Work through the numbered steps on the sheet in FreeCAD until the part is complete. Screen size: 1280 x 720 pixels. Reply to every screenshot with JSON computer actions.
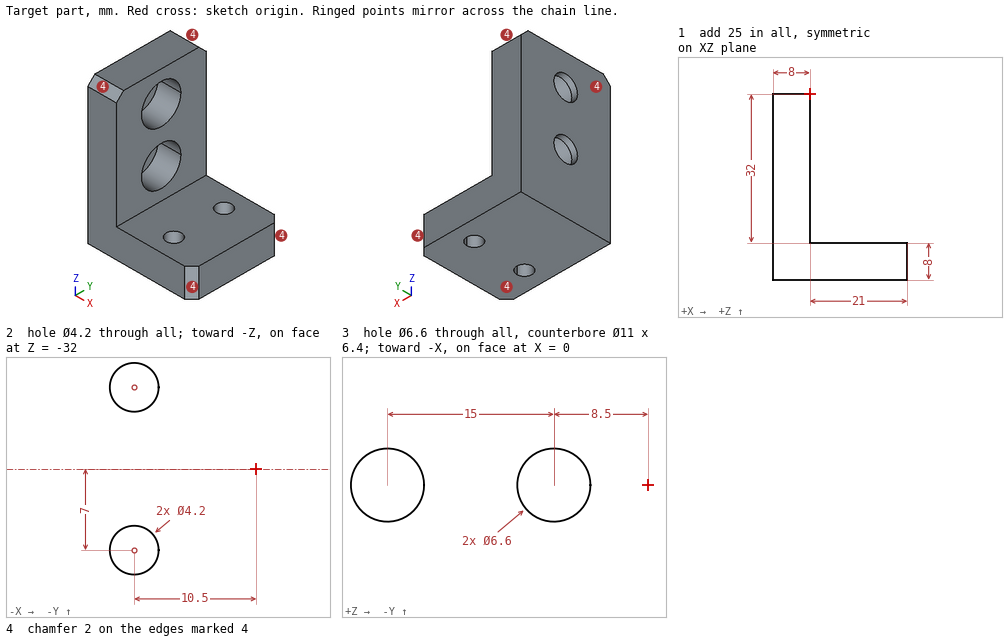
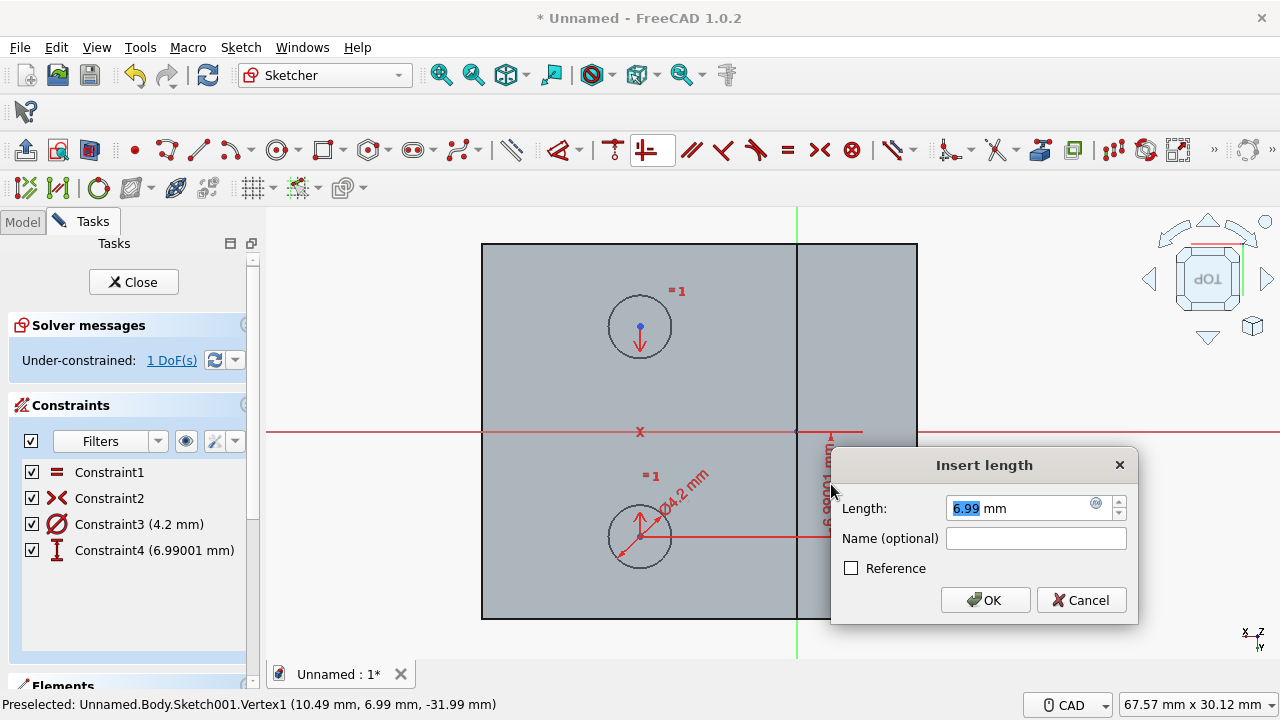
{"action": "type", "text": "7"}
{"action": "key", "text": "Return"}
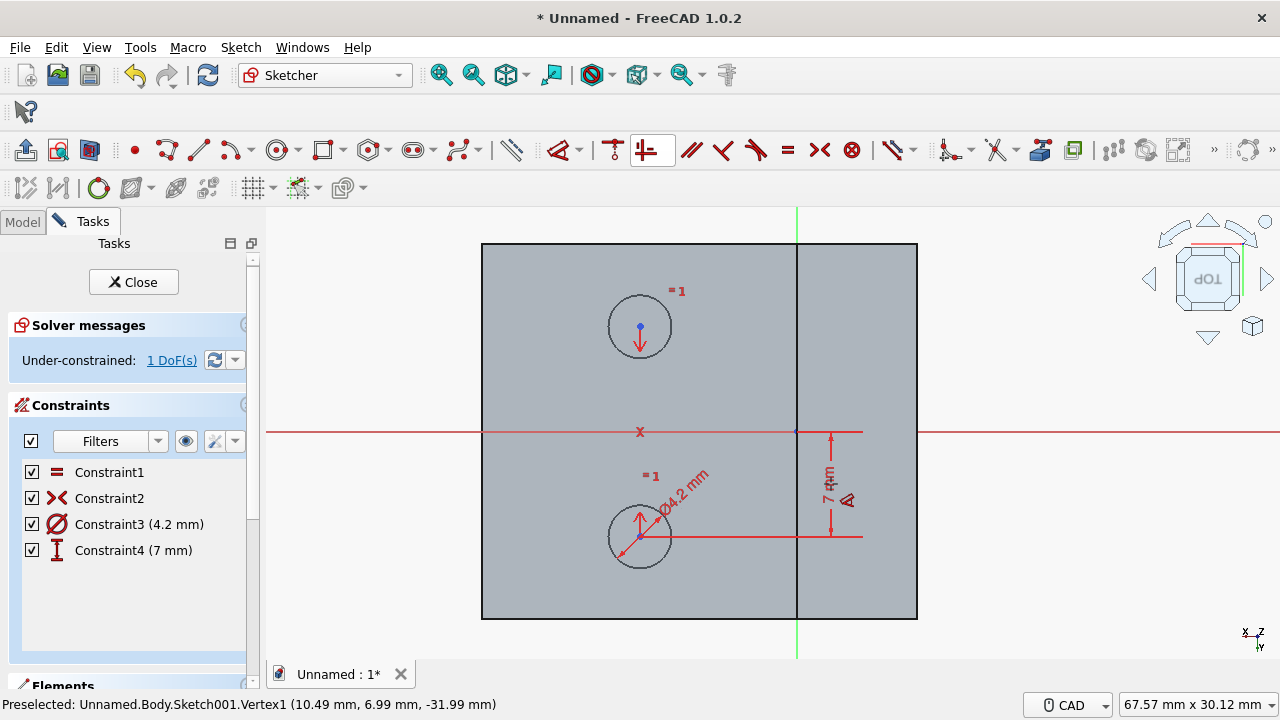
{"action": "left_click", "coordinate": [640, 537]}
{"action": "left_click", "coordinate": [719, 571]}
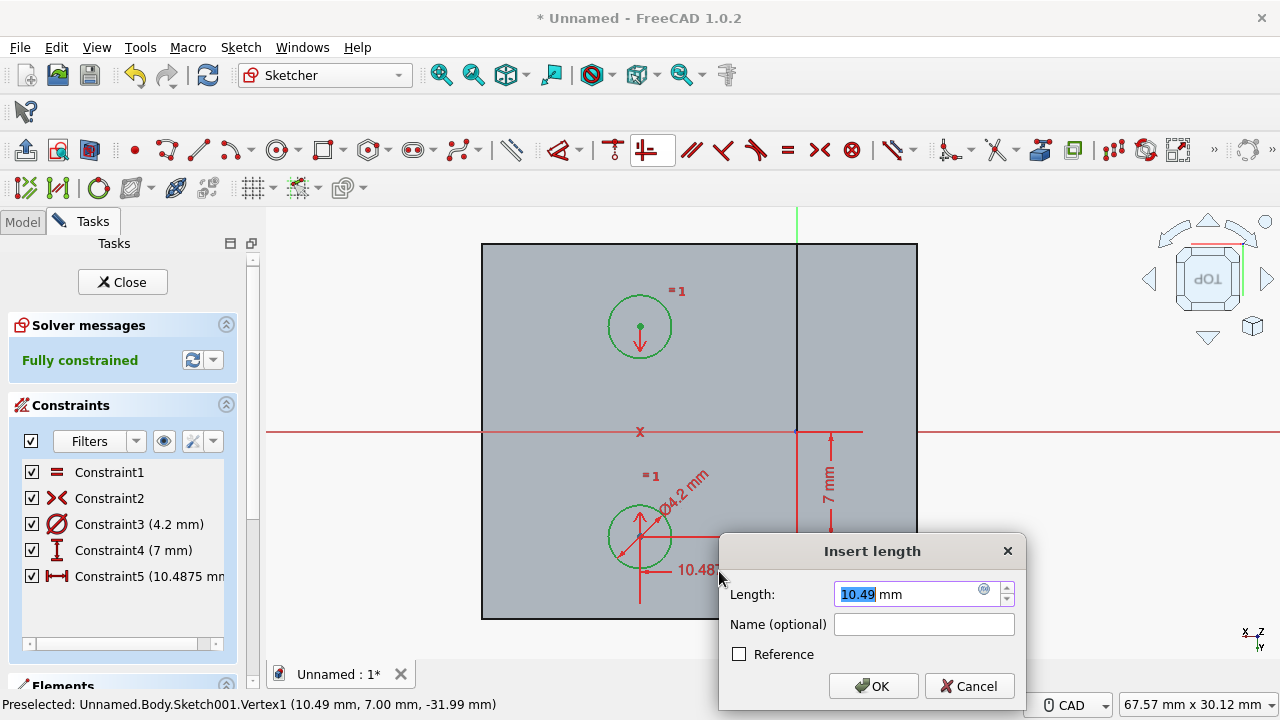
{"action": "type", "text": "10.5"}
{"action": "key", "text": "Return"}
{"action": "key", "text": "Escape"}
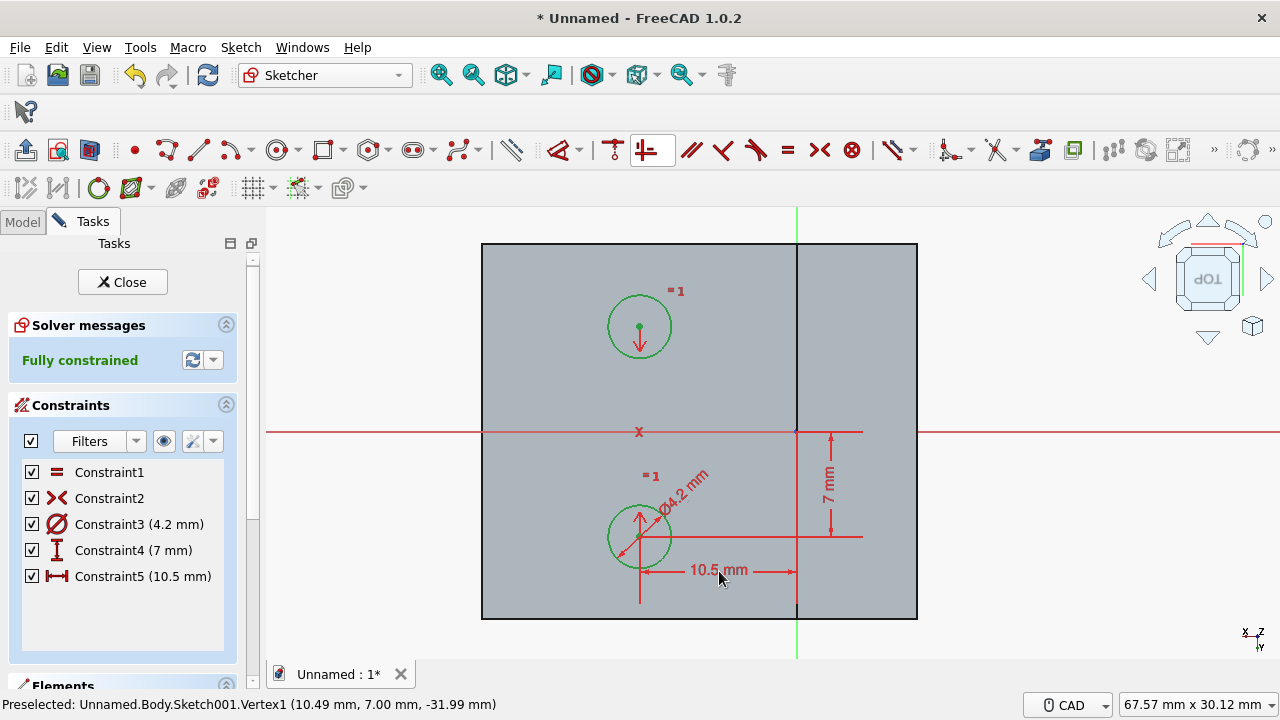
{"action": "left_click", "coordinate": [123, 282]}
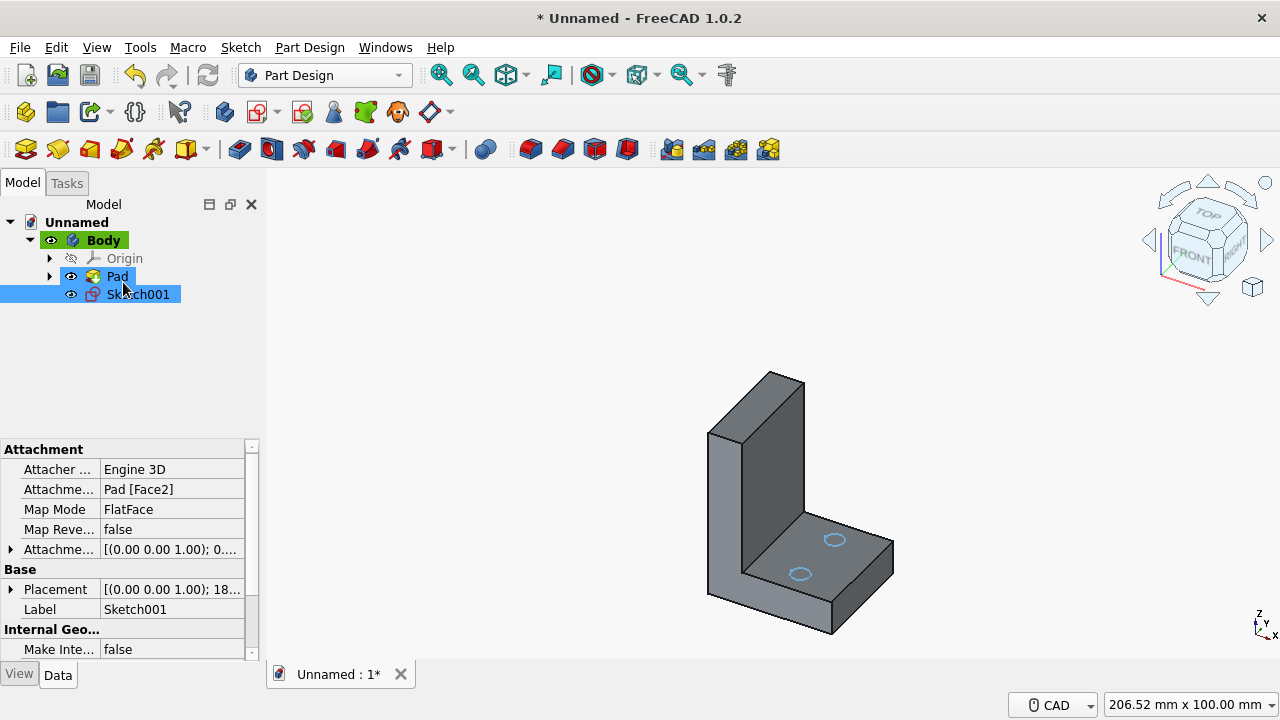
{"action": "left_click", "coordinate": [272, 150]}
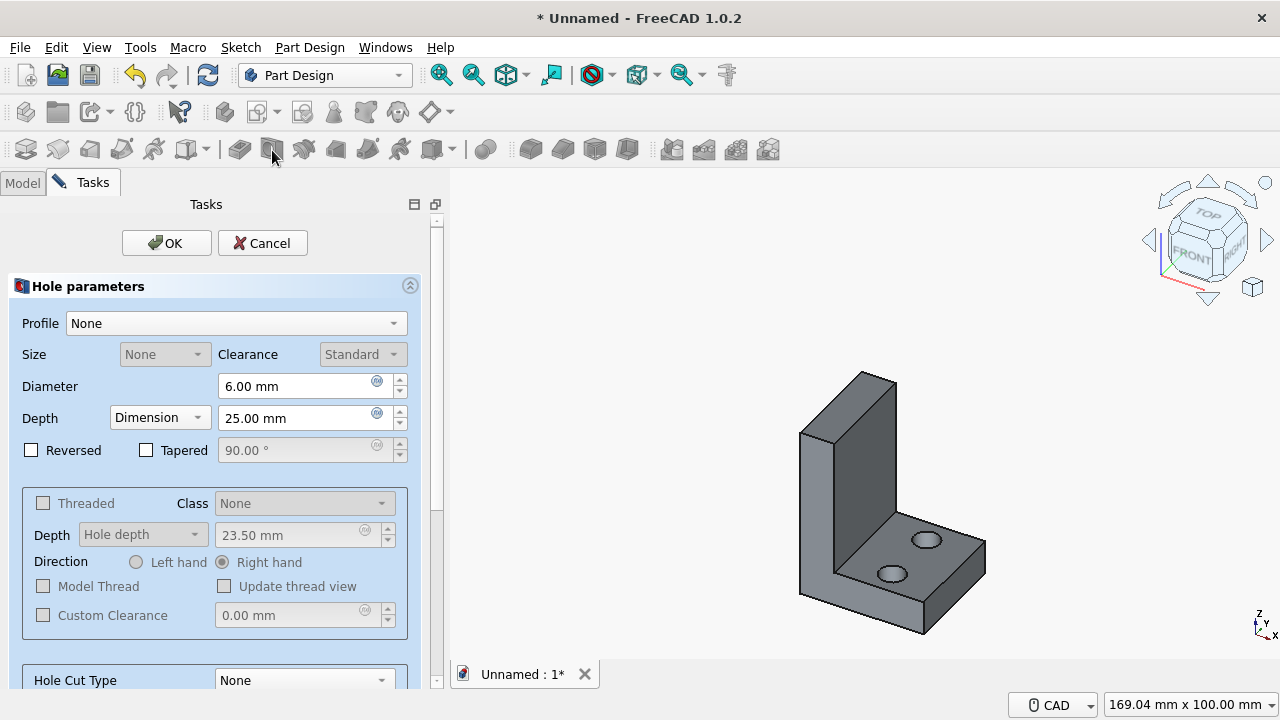
{"action": "triple_click", "coordinate": [305, 386]}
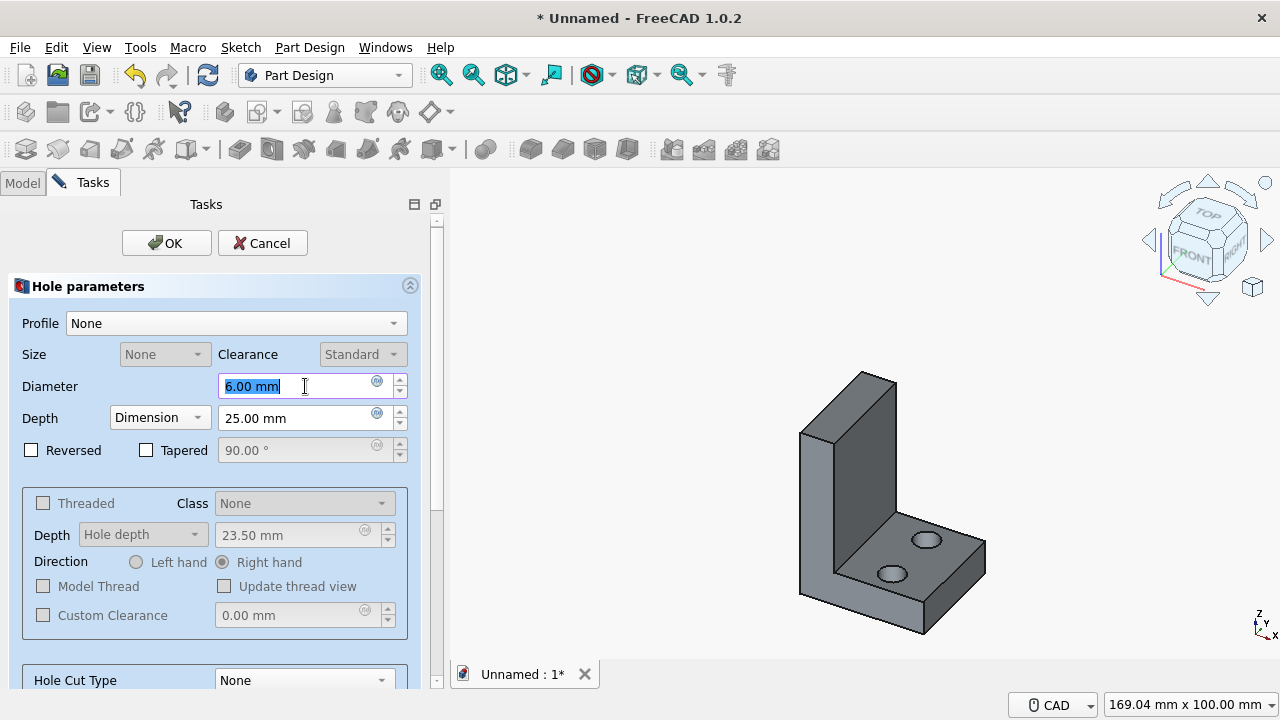
{"action": "type", "text": "4.2"}
{"action": "key", "text": "Tab"}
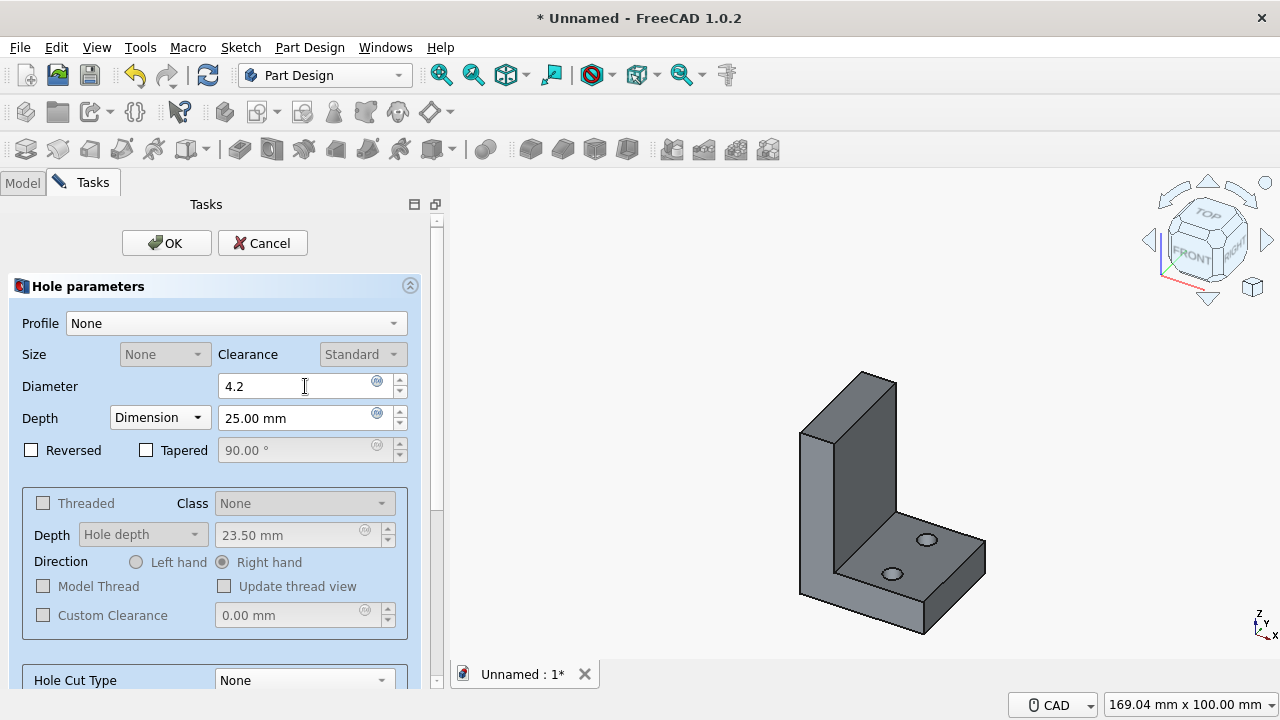
{"action": "left_click", "coordinate": [161, 418]}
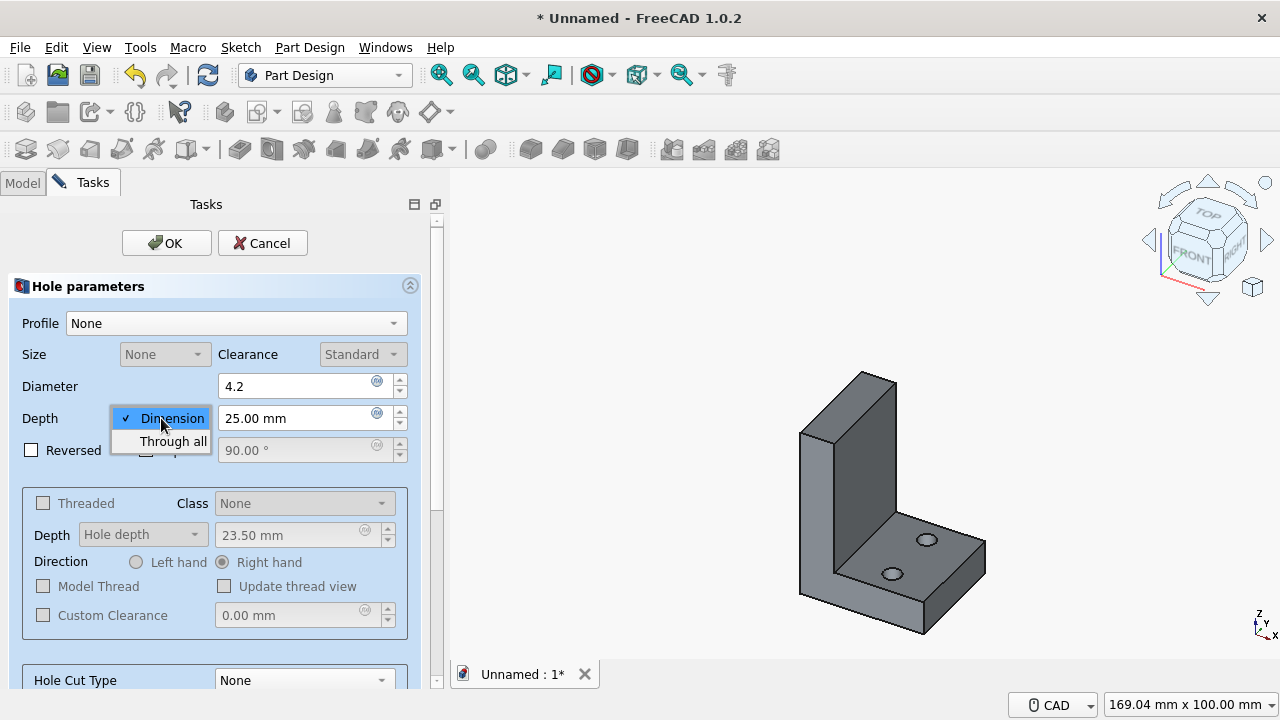
{"action": "left_click", "coordinate": [160, 442]}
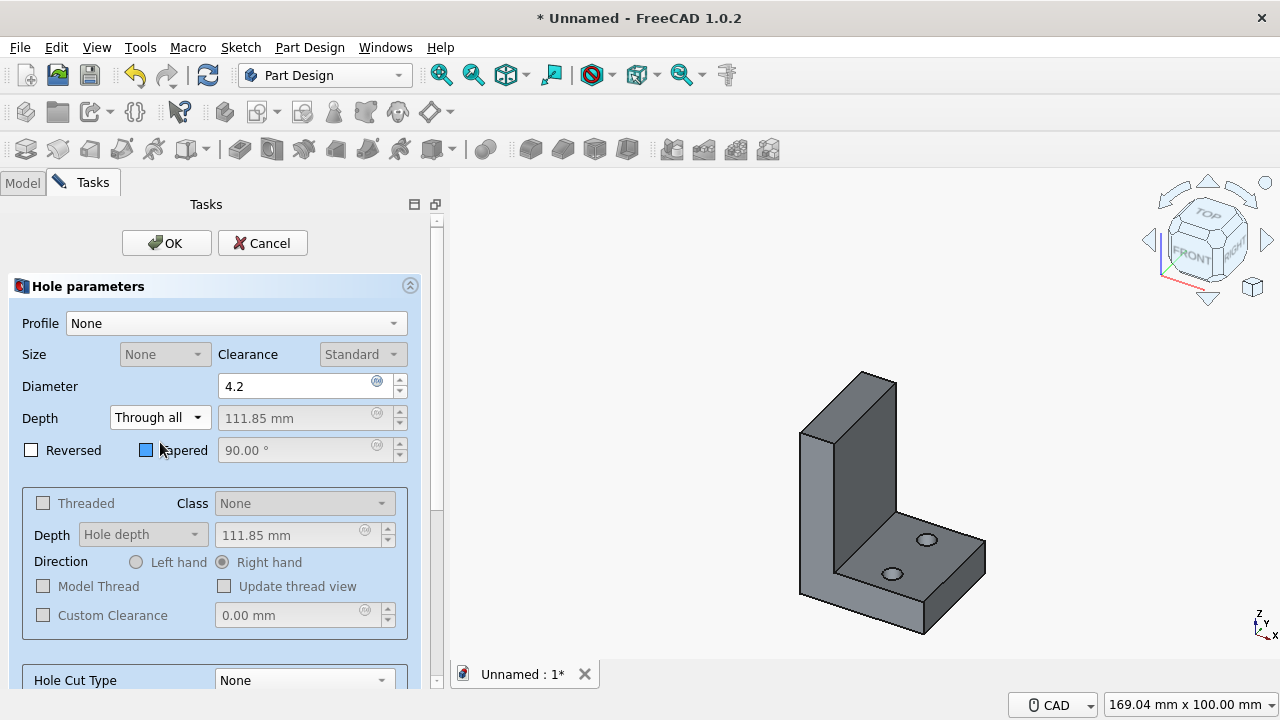
{"action": "left_click", "coordinate": [167, 243]}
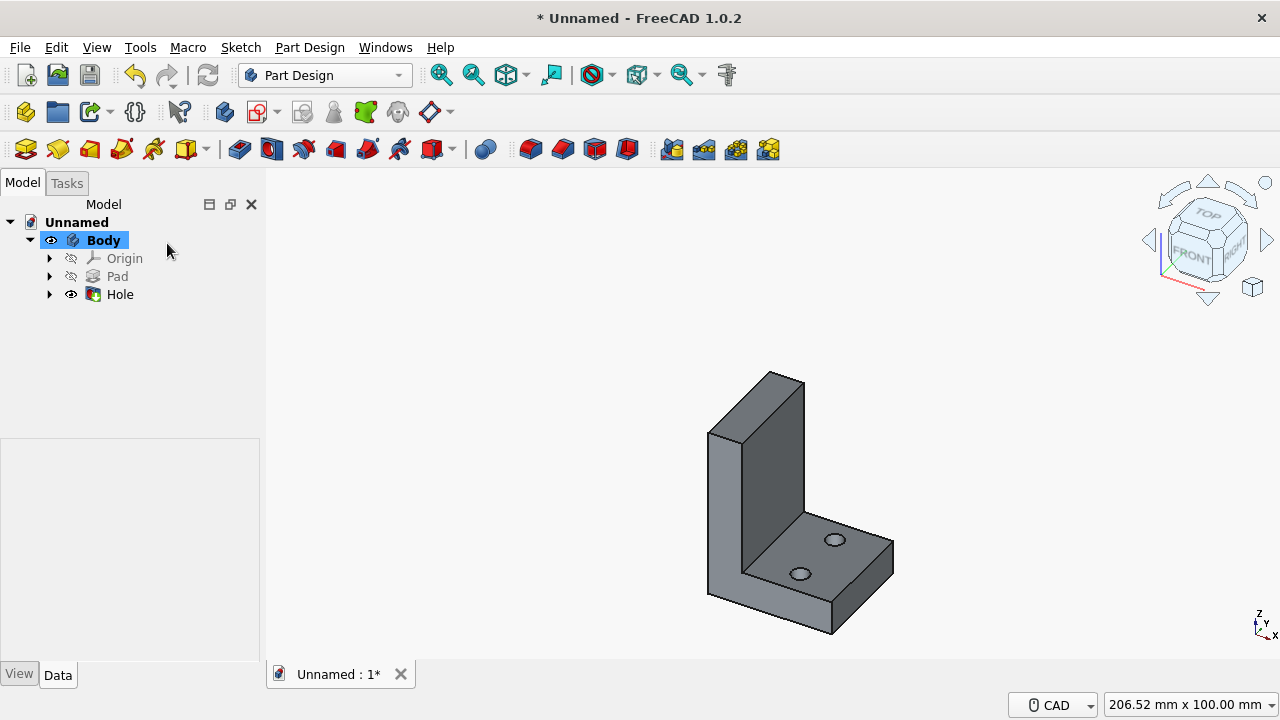
{"action": "left_click", "coordinate": [773, 477]}